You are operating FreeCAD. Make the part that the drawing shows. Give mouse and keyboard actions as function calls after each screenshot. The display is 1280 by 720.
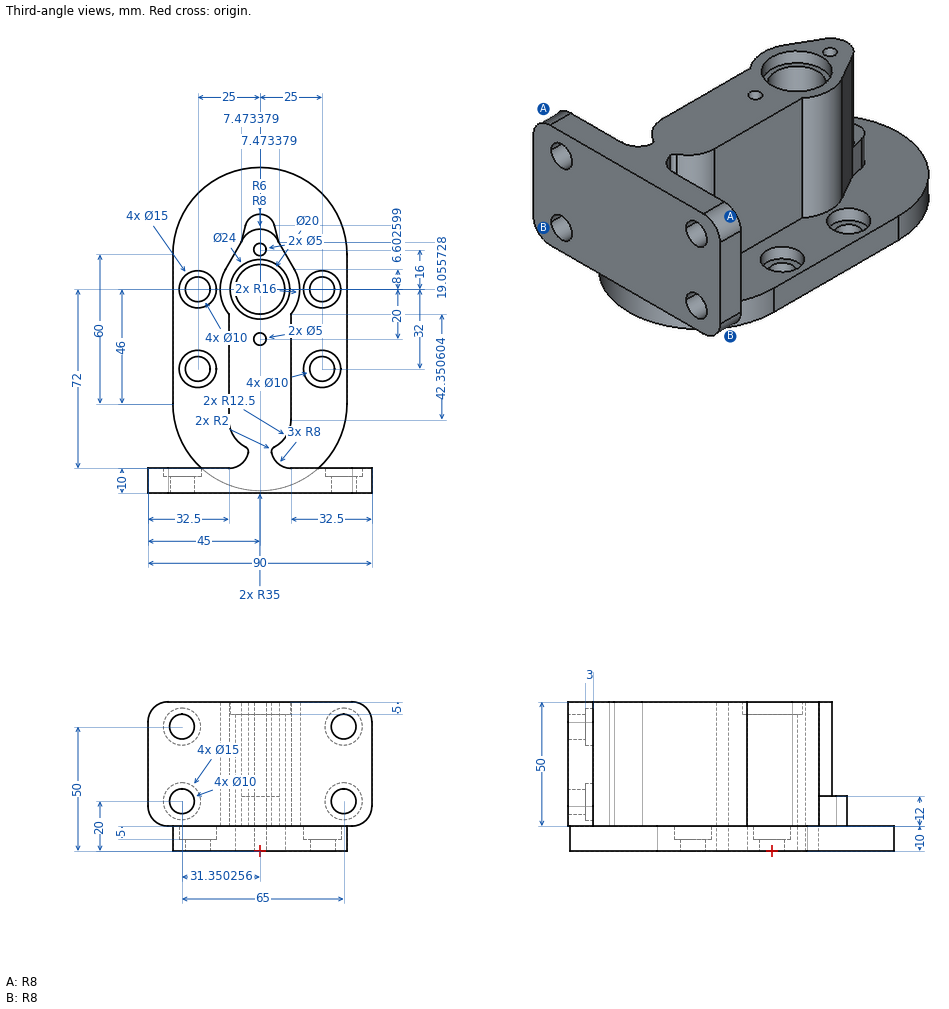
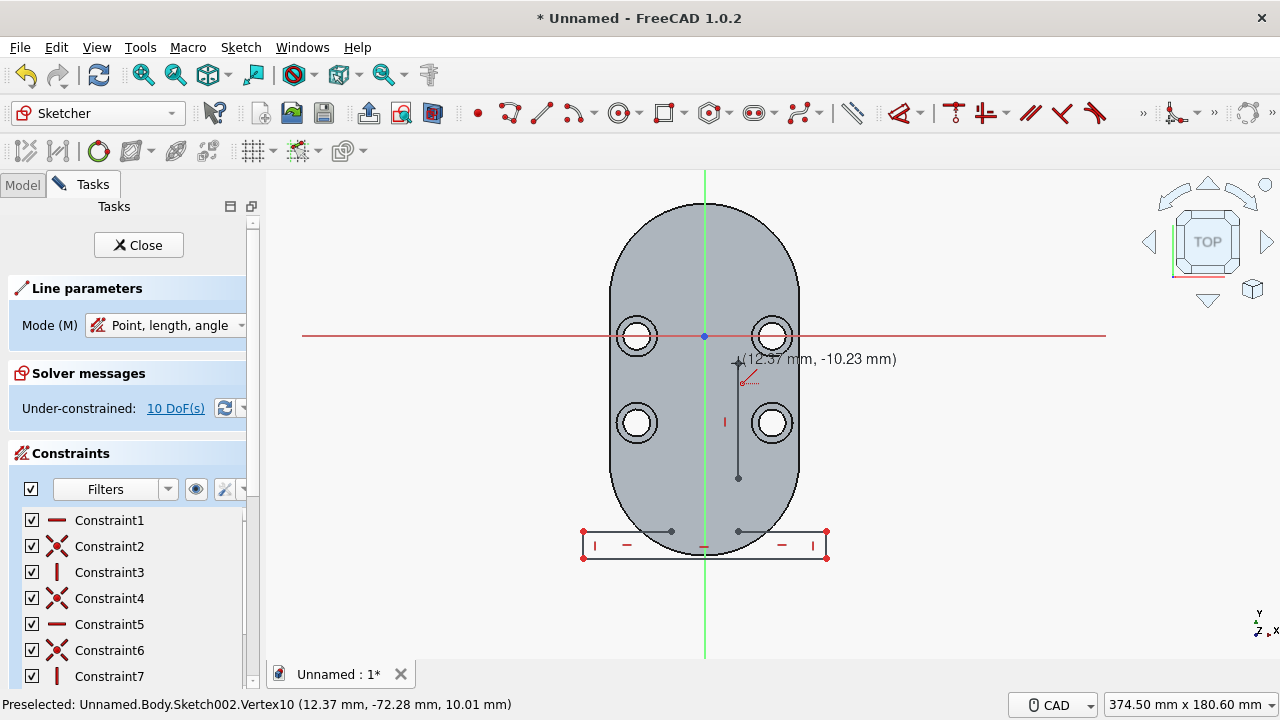
click(742, 315)
click(725, 285)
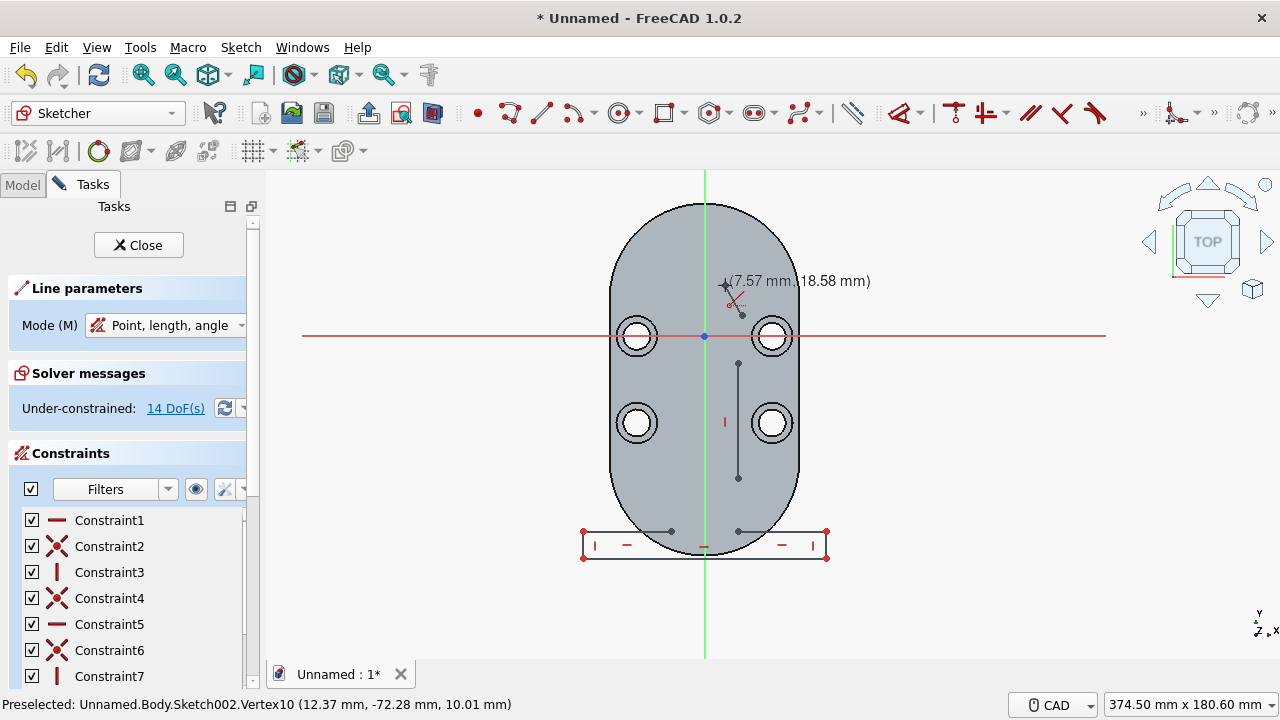
click(684, 285)
click(667, 315)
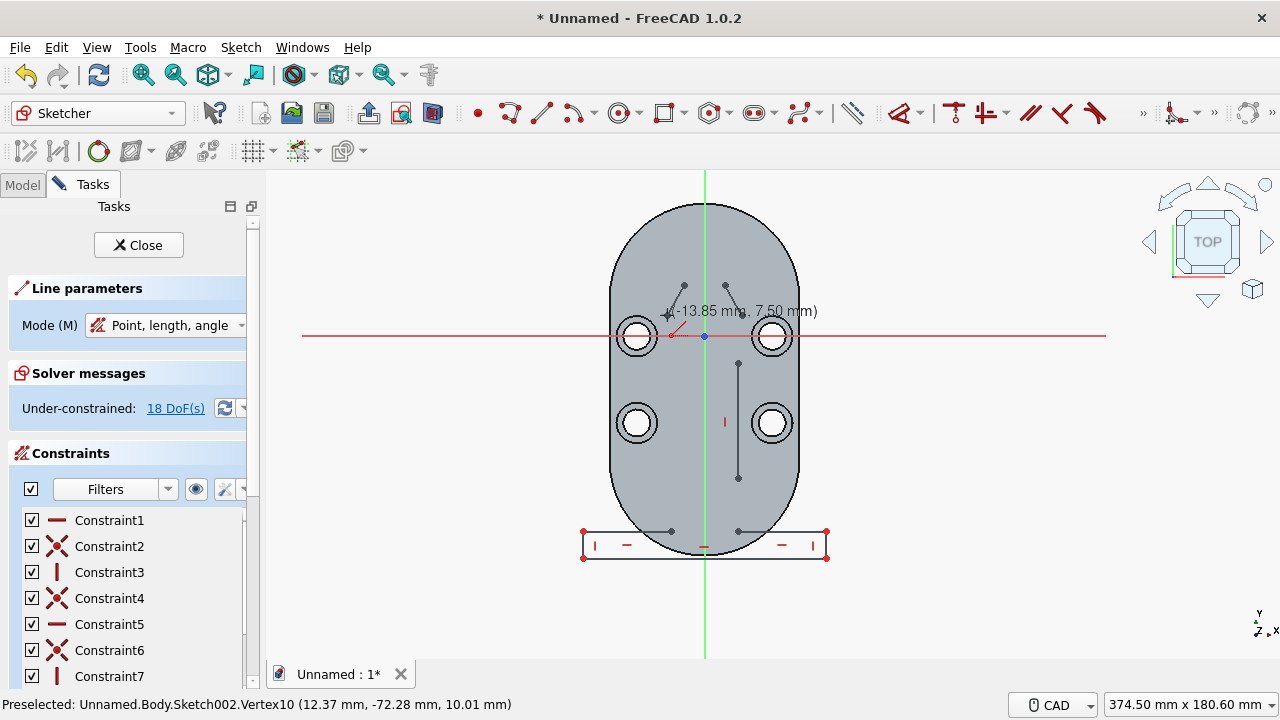
click(671, 363)
click(671, 478)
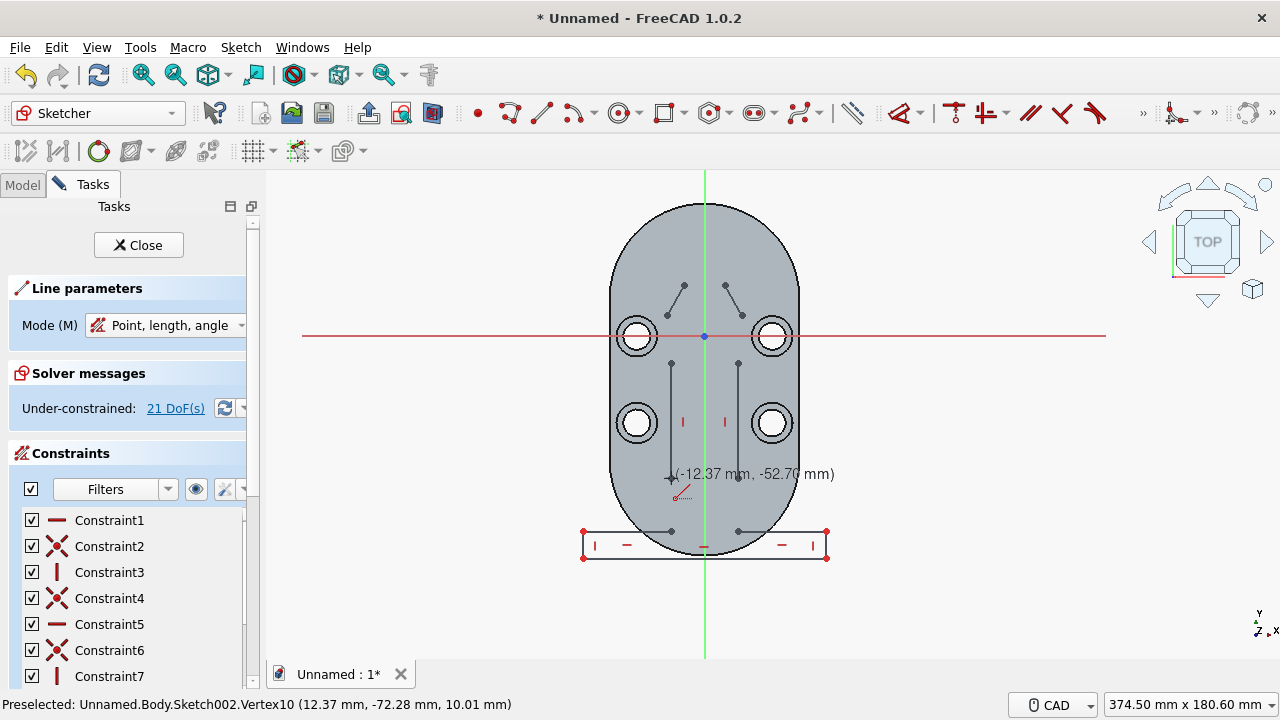
click(596, 114)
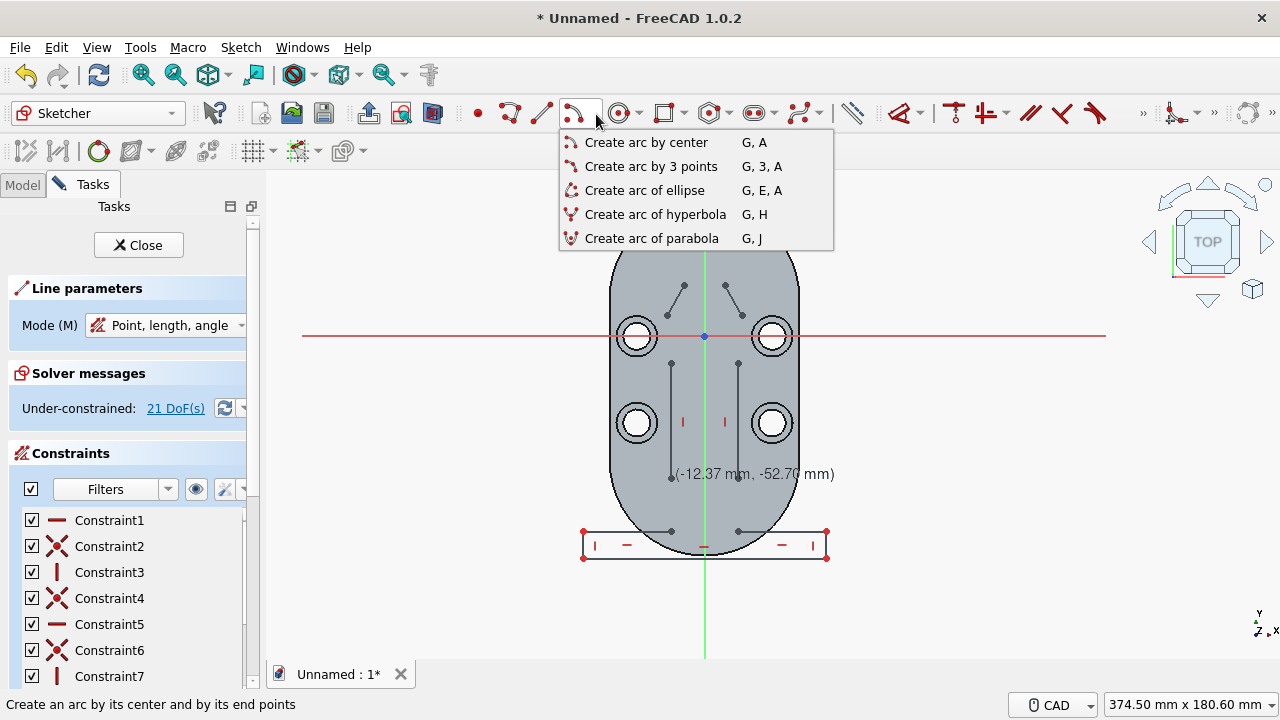
click(696, 166)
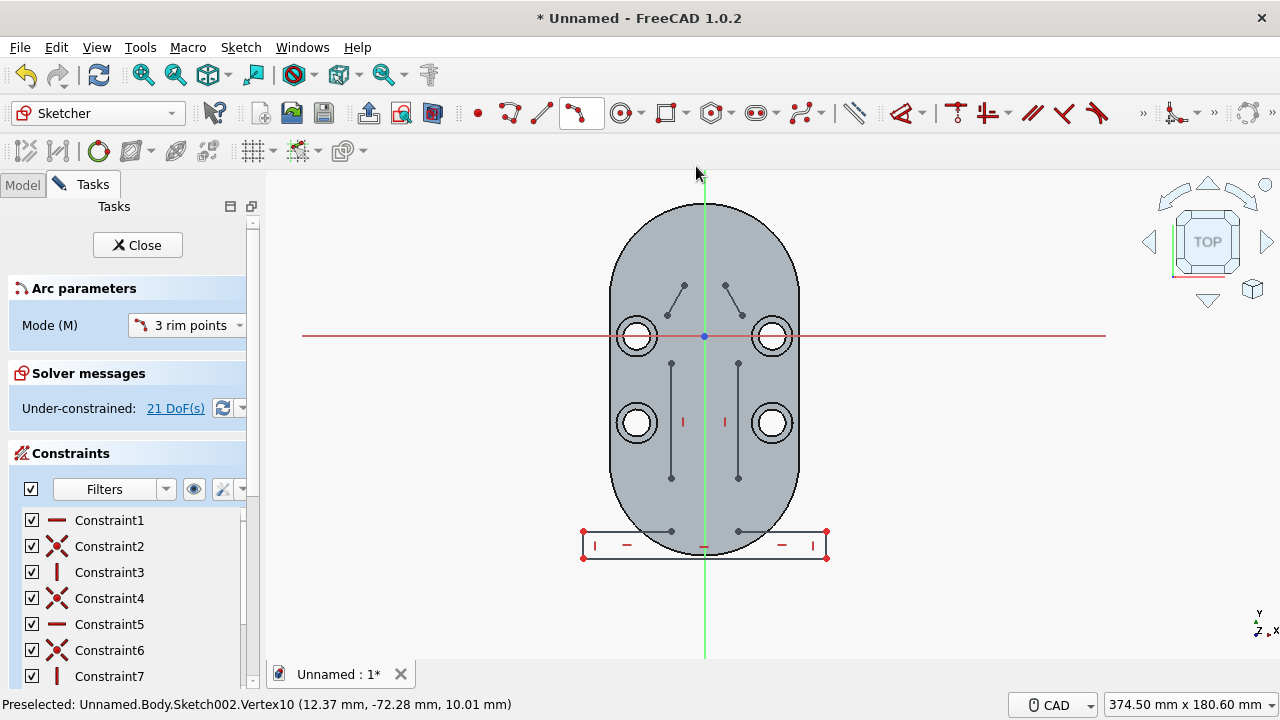
click(738, 532)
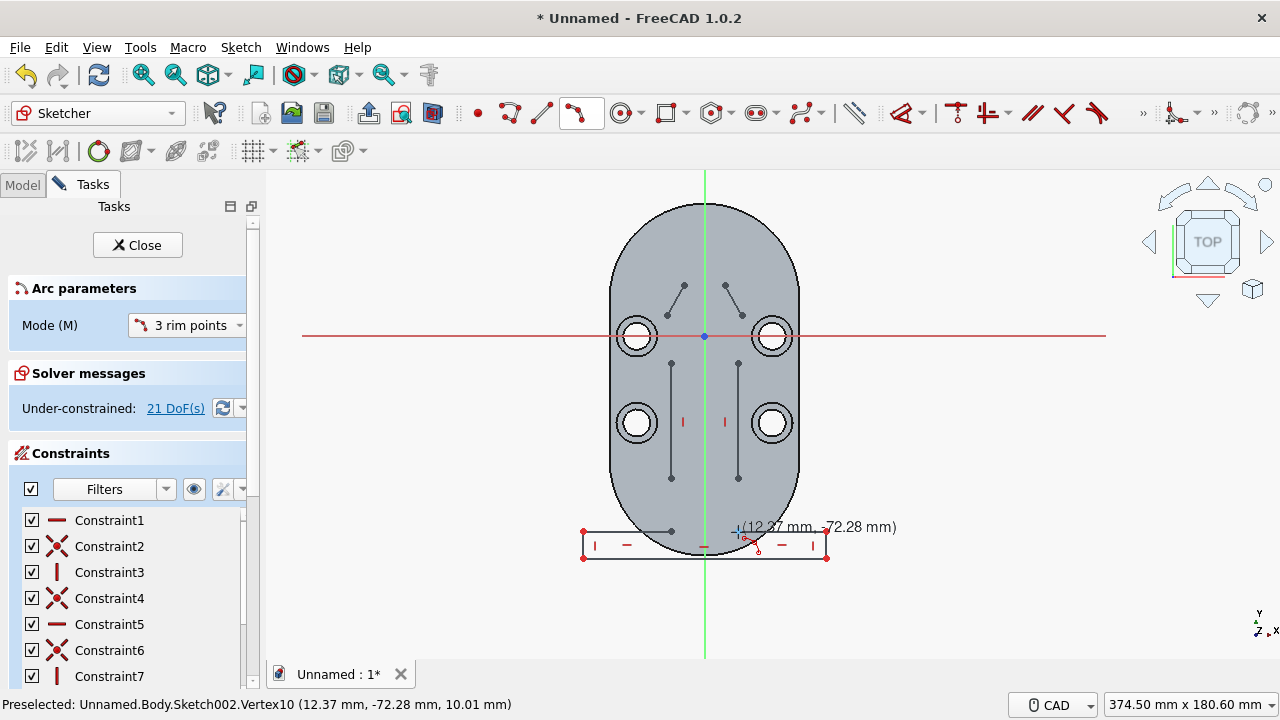
scroll(717, 514, up, 2)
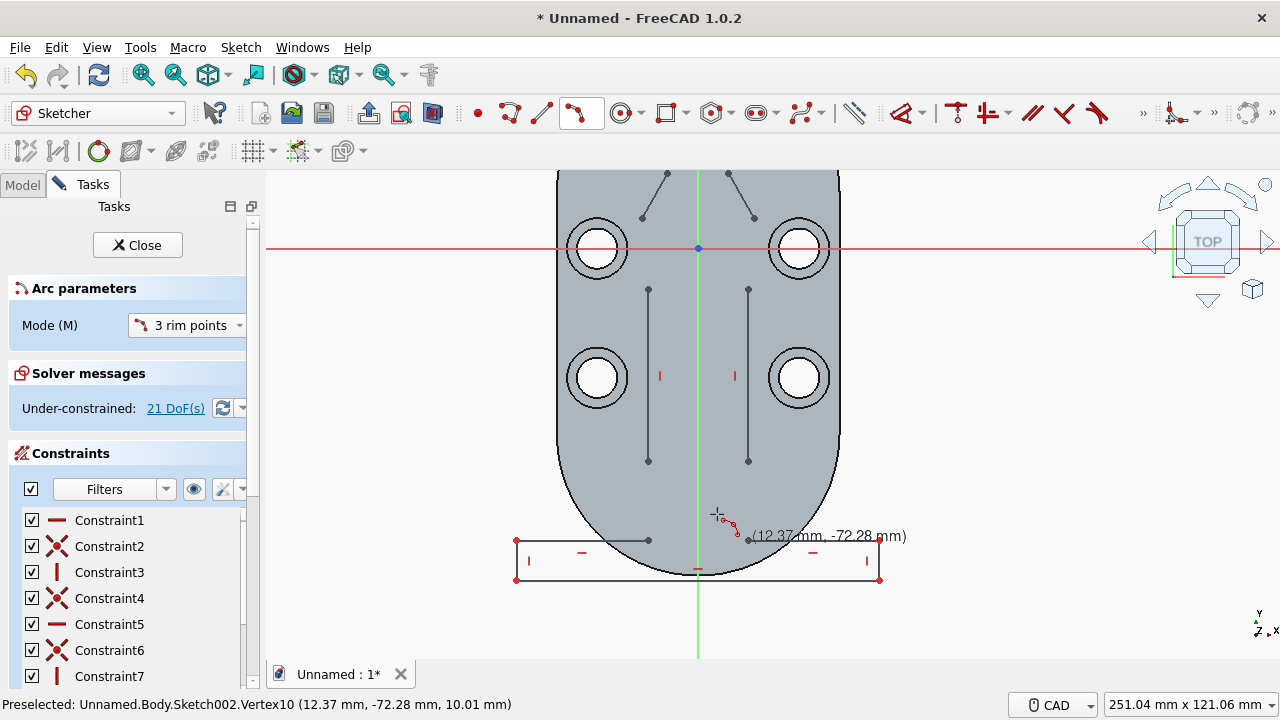
click(717, 514)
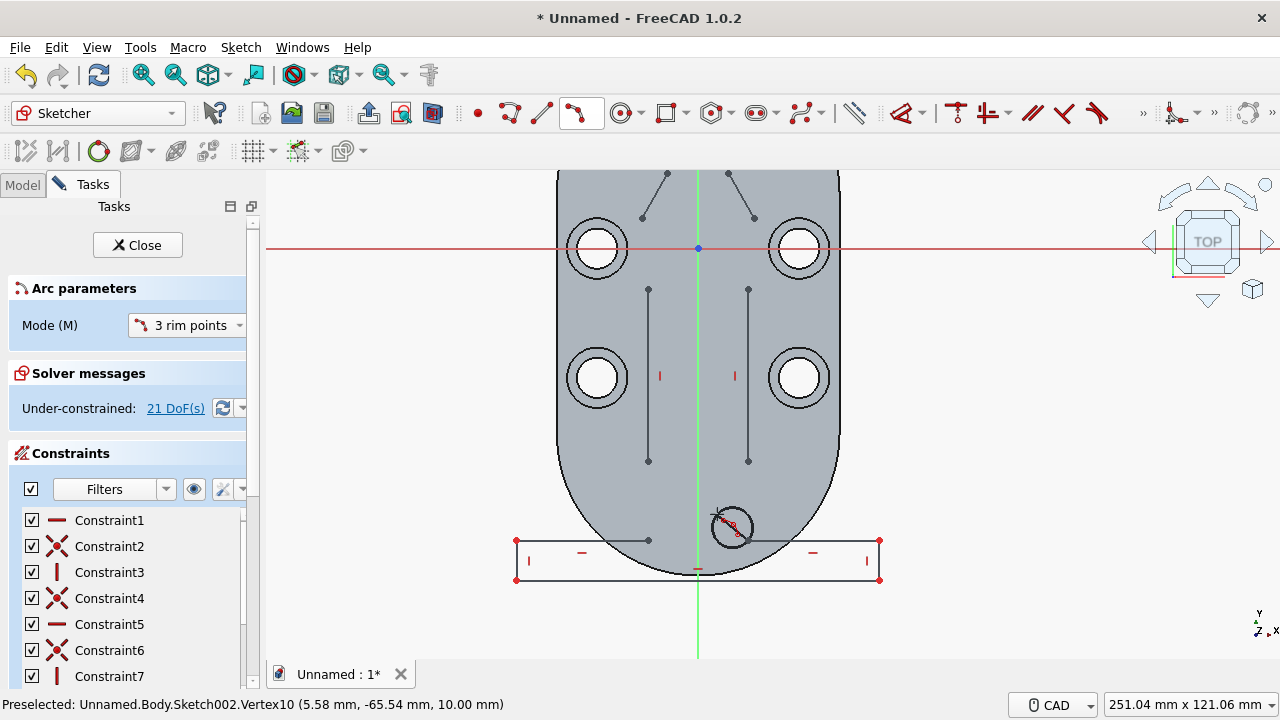
scroll(728, 532, up, 4)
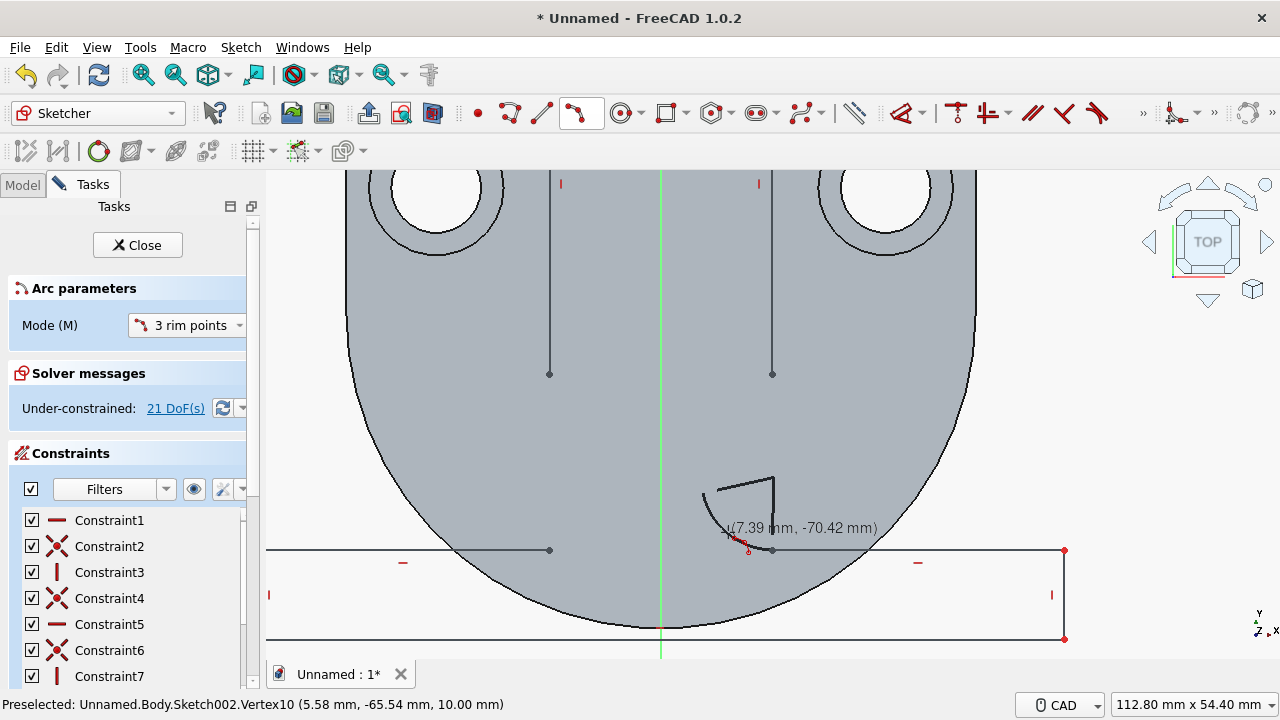
click(728, 531)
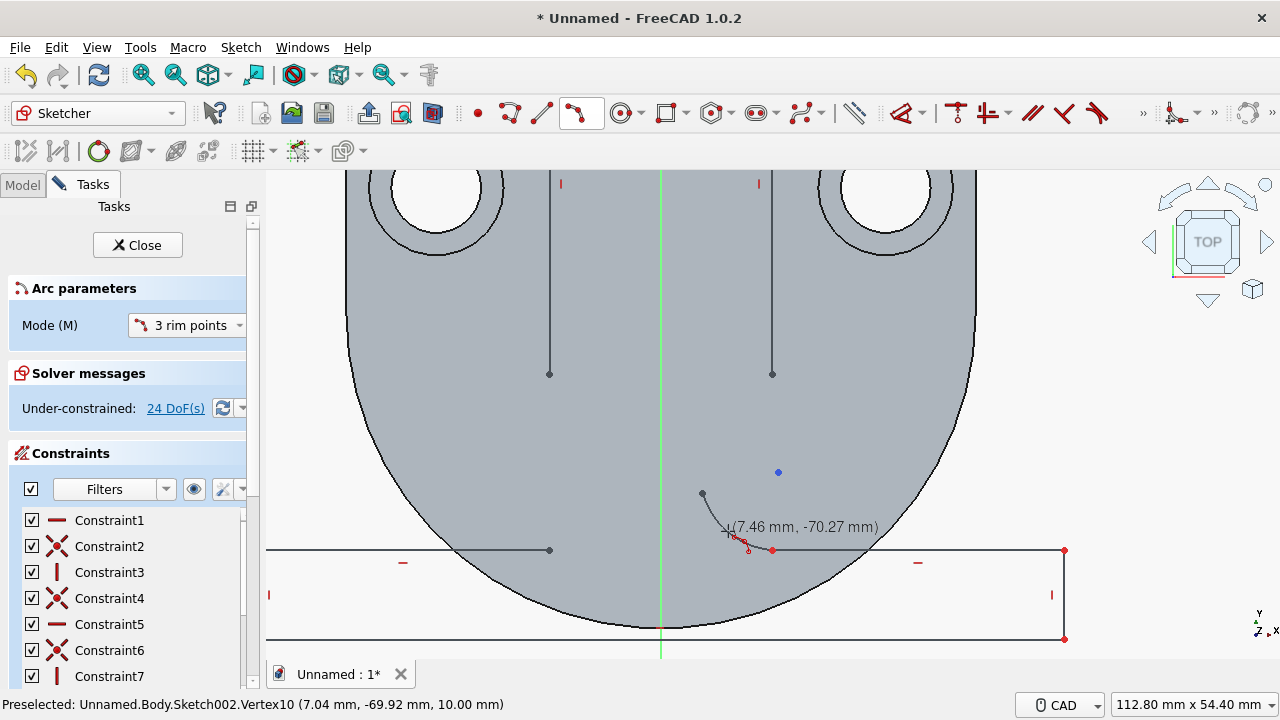
click(703, 493)
click(712, 471)